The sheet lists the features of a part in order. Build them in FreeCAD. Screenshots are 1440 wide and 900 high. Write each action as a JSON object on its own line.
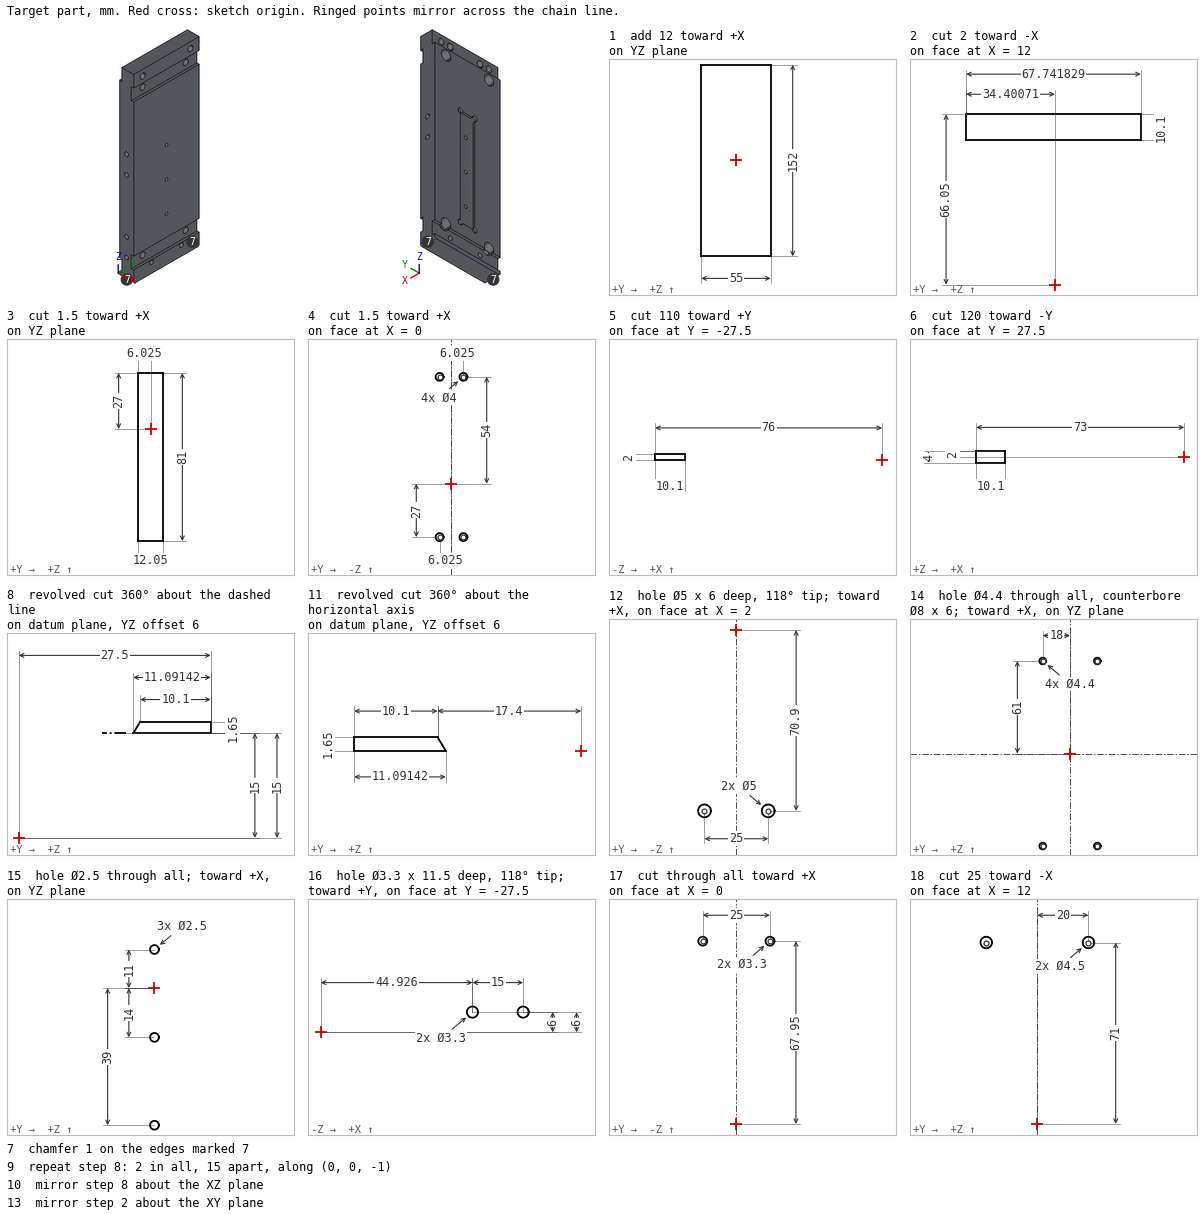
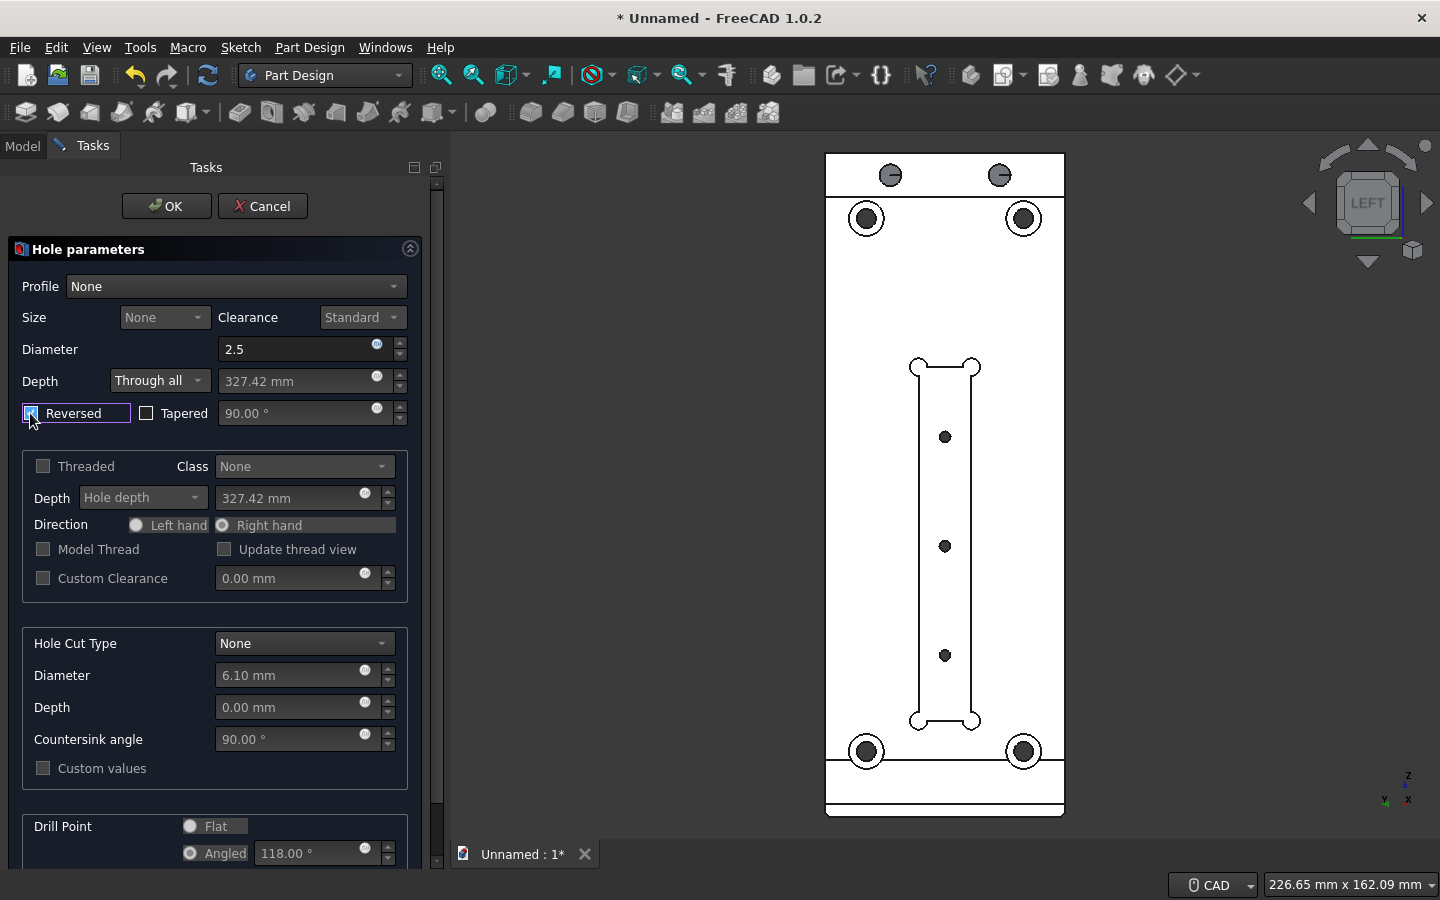
{"action": "left_click", "coordinate": [167, 206]}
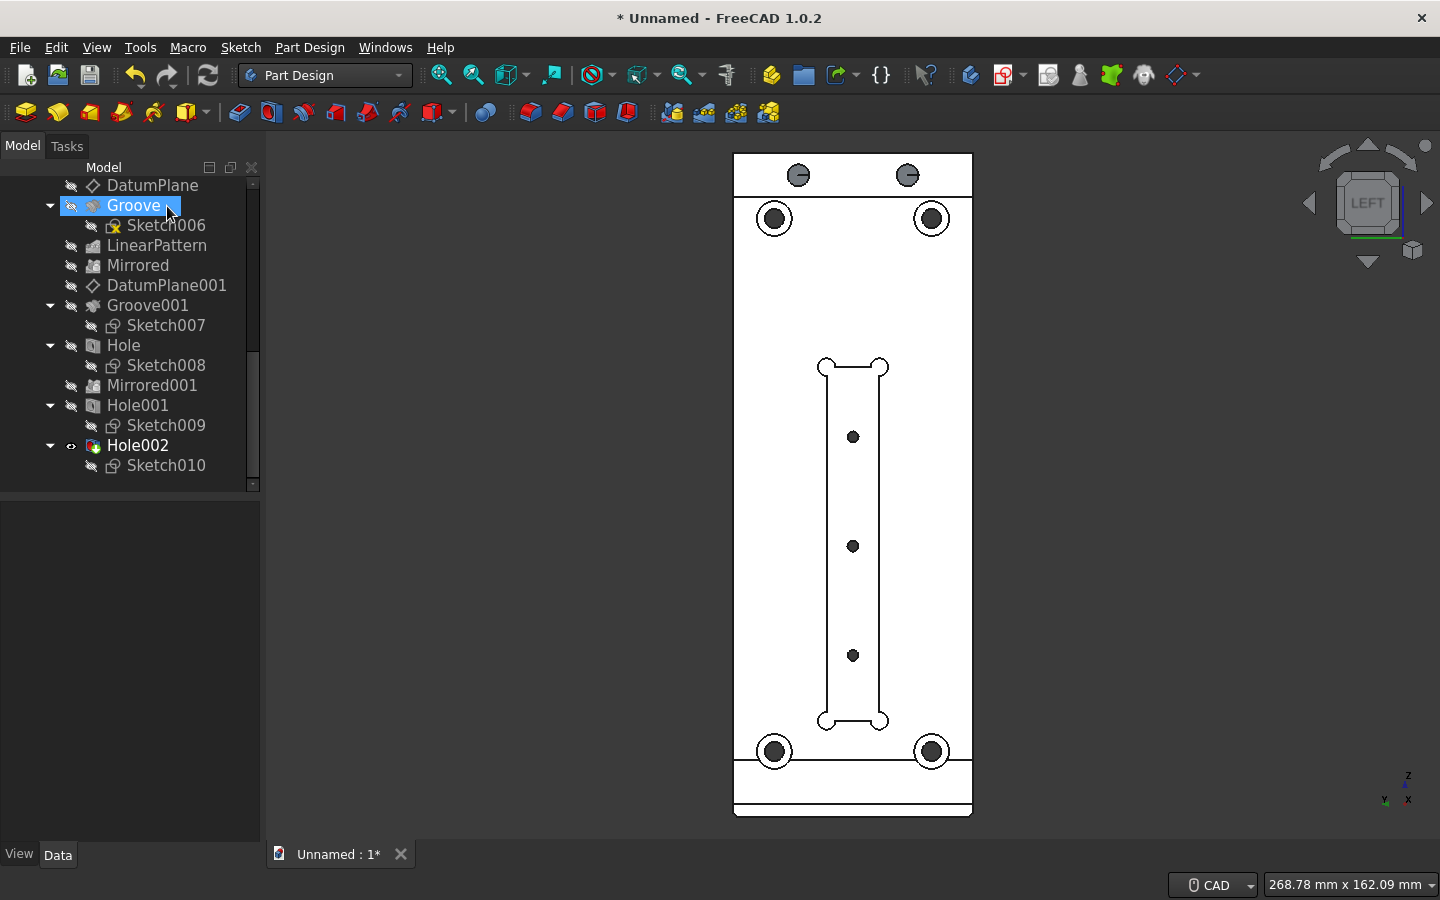
{"action": "key", "text": "0"}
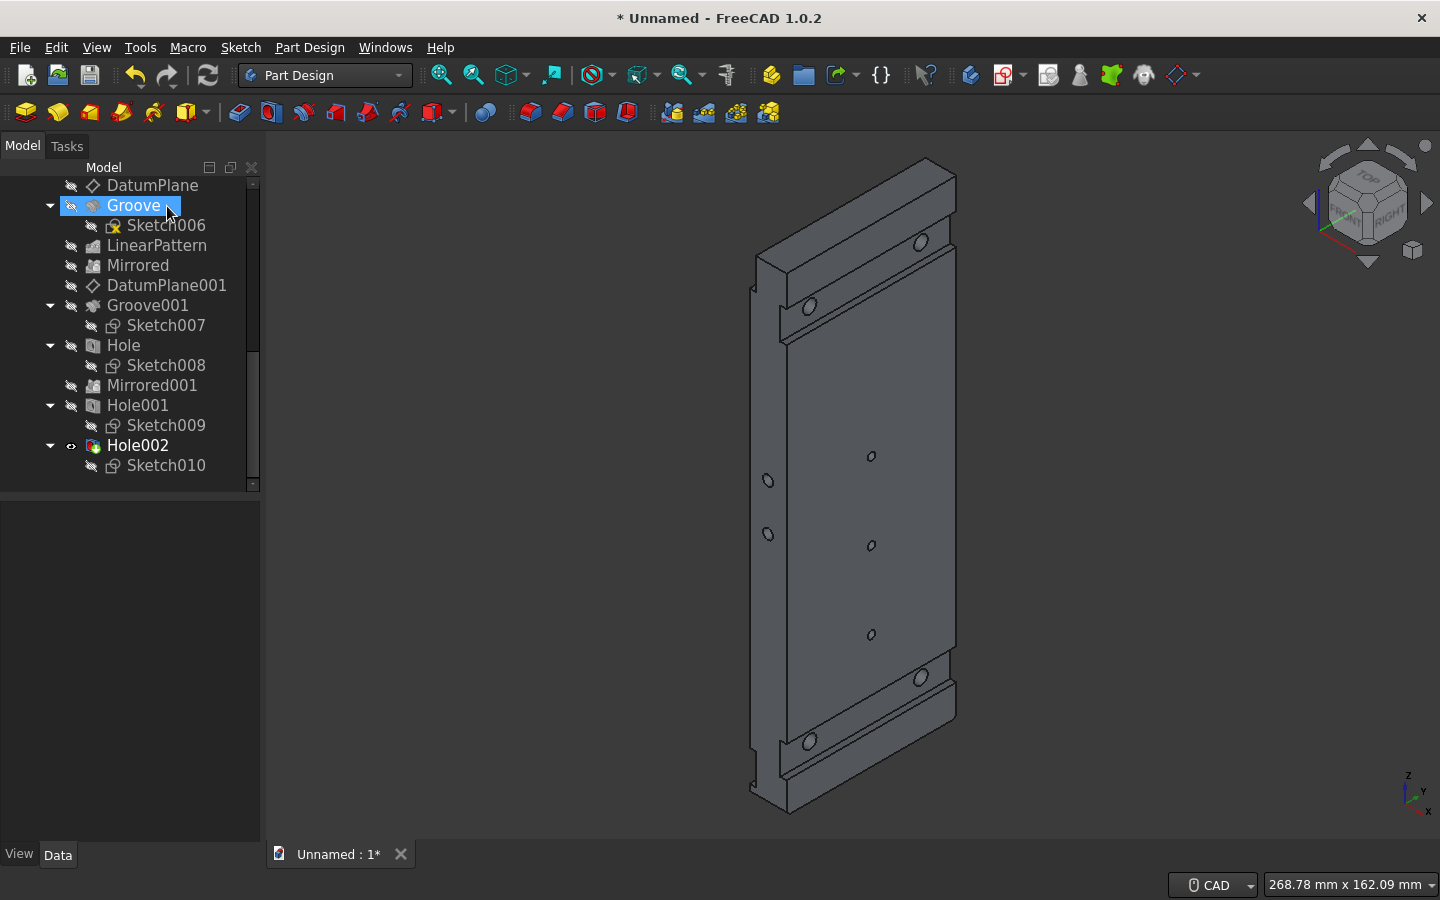
{"action": "left_click", "coordinate": [768, 685]}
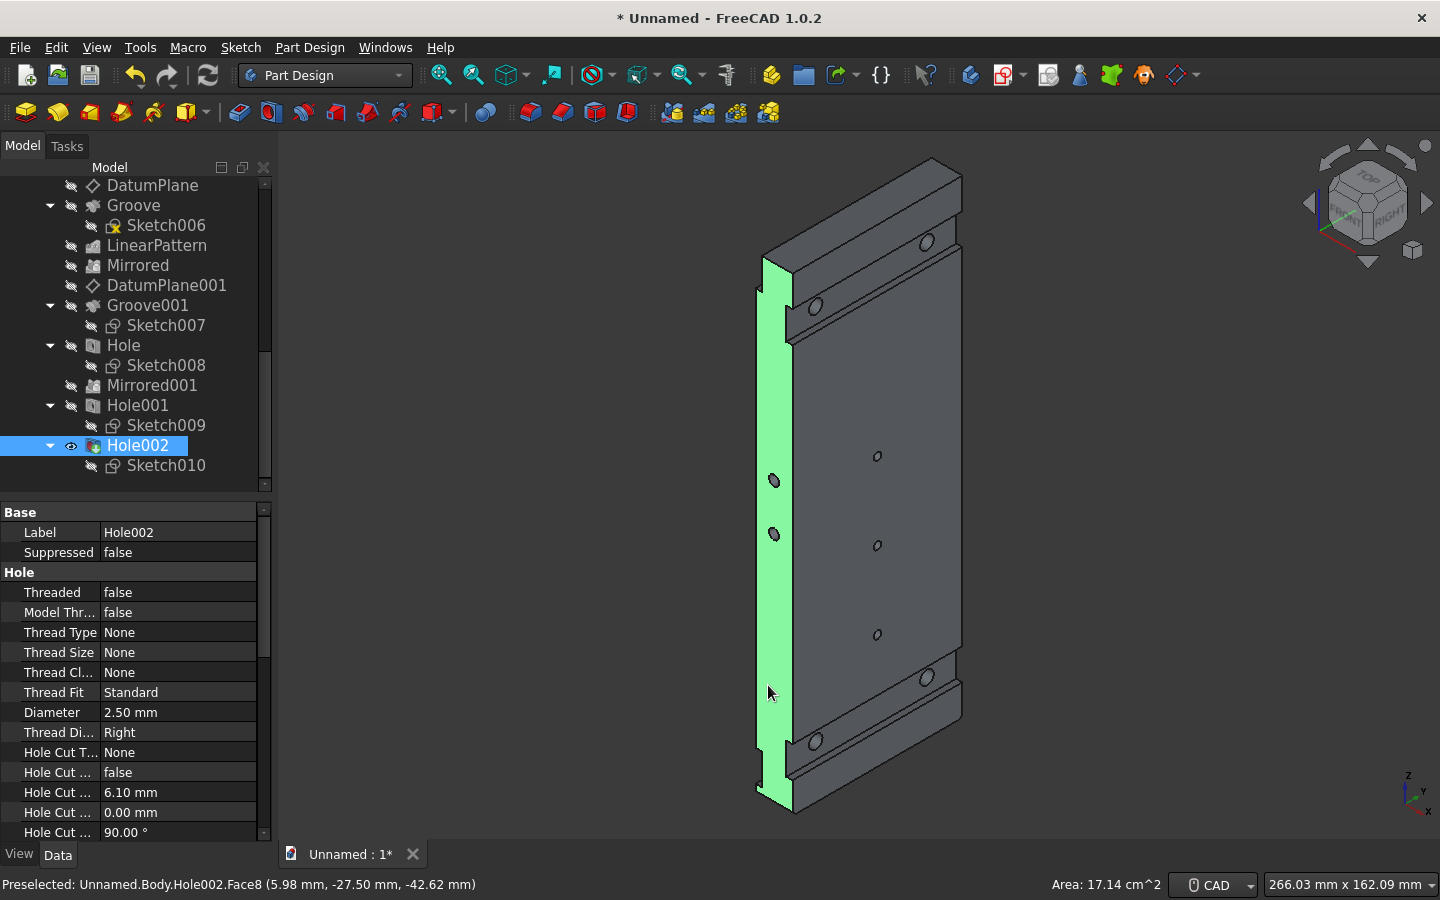
{"action": "left_click", "coordinate": [1004, 76]}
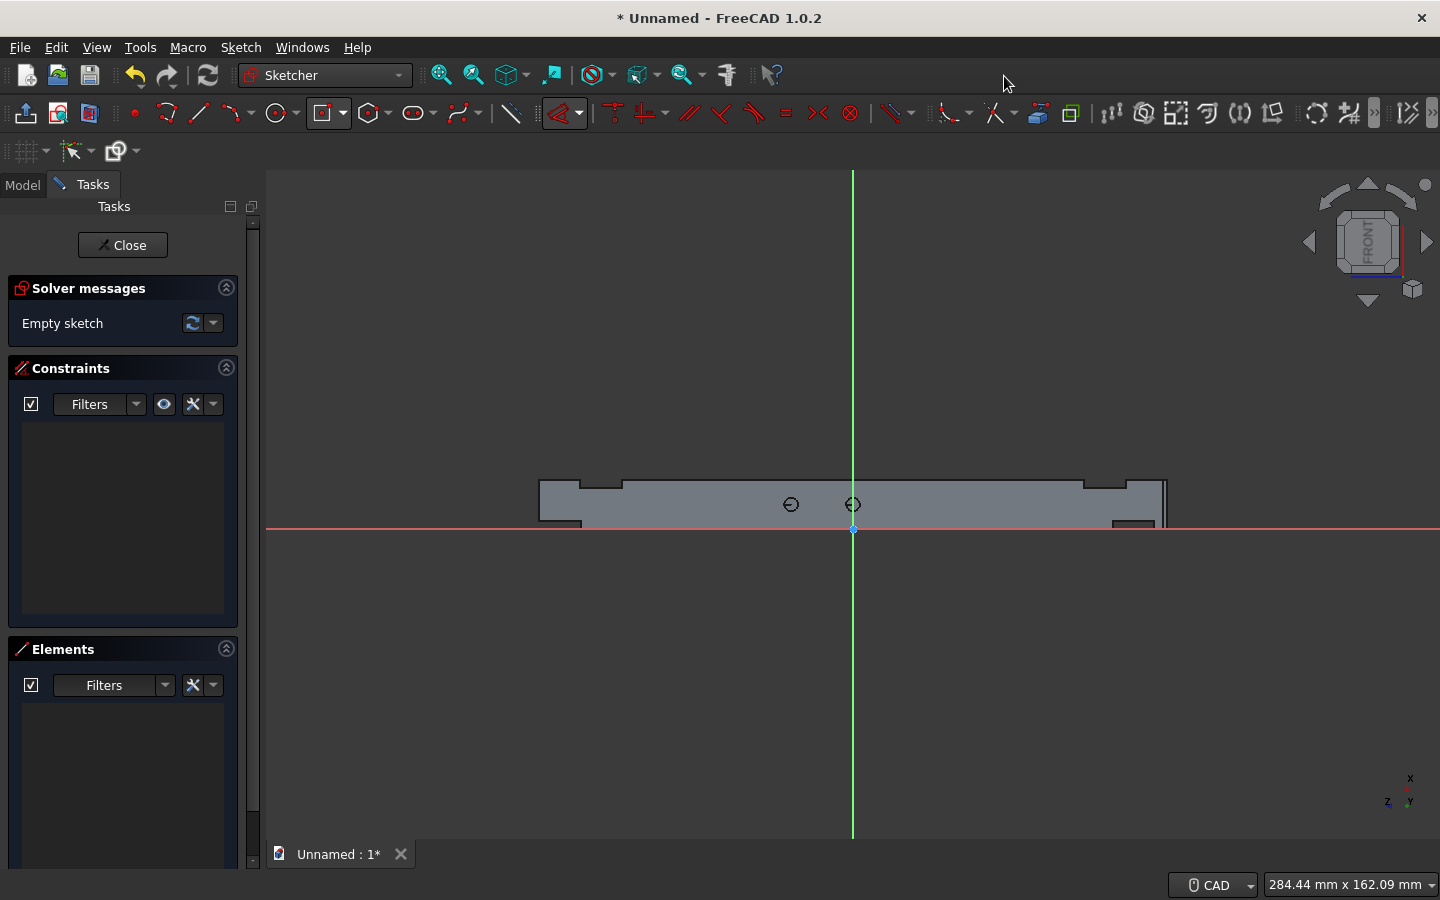
{"action": "scroll", "coordinate": [1105, 505], "scroll_direction": "up", "scroll_amount": 11}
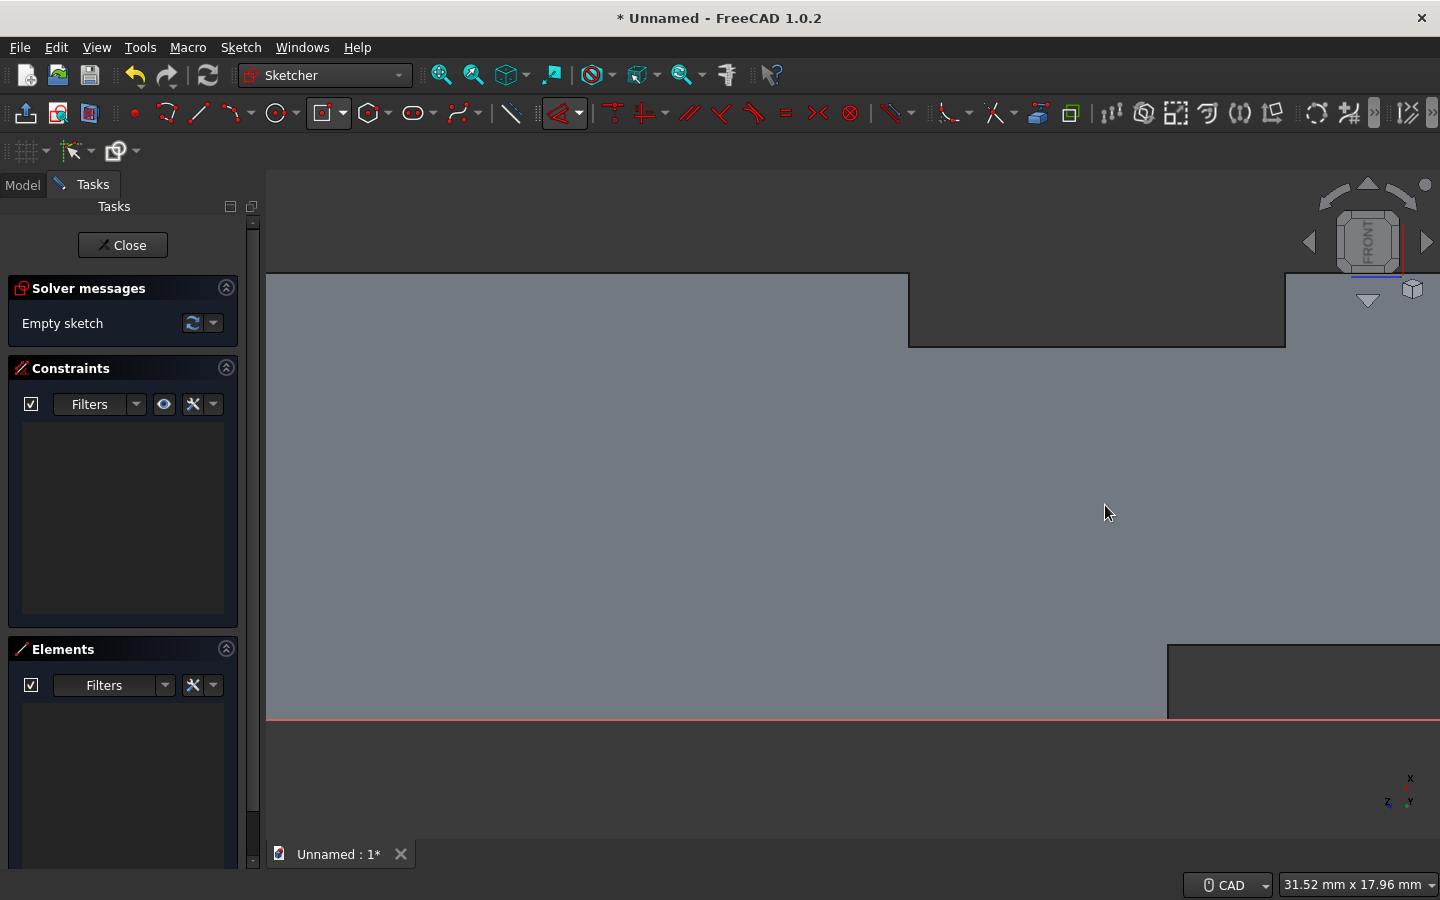
{"action": "left_click", "coordinate": [276, 114]}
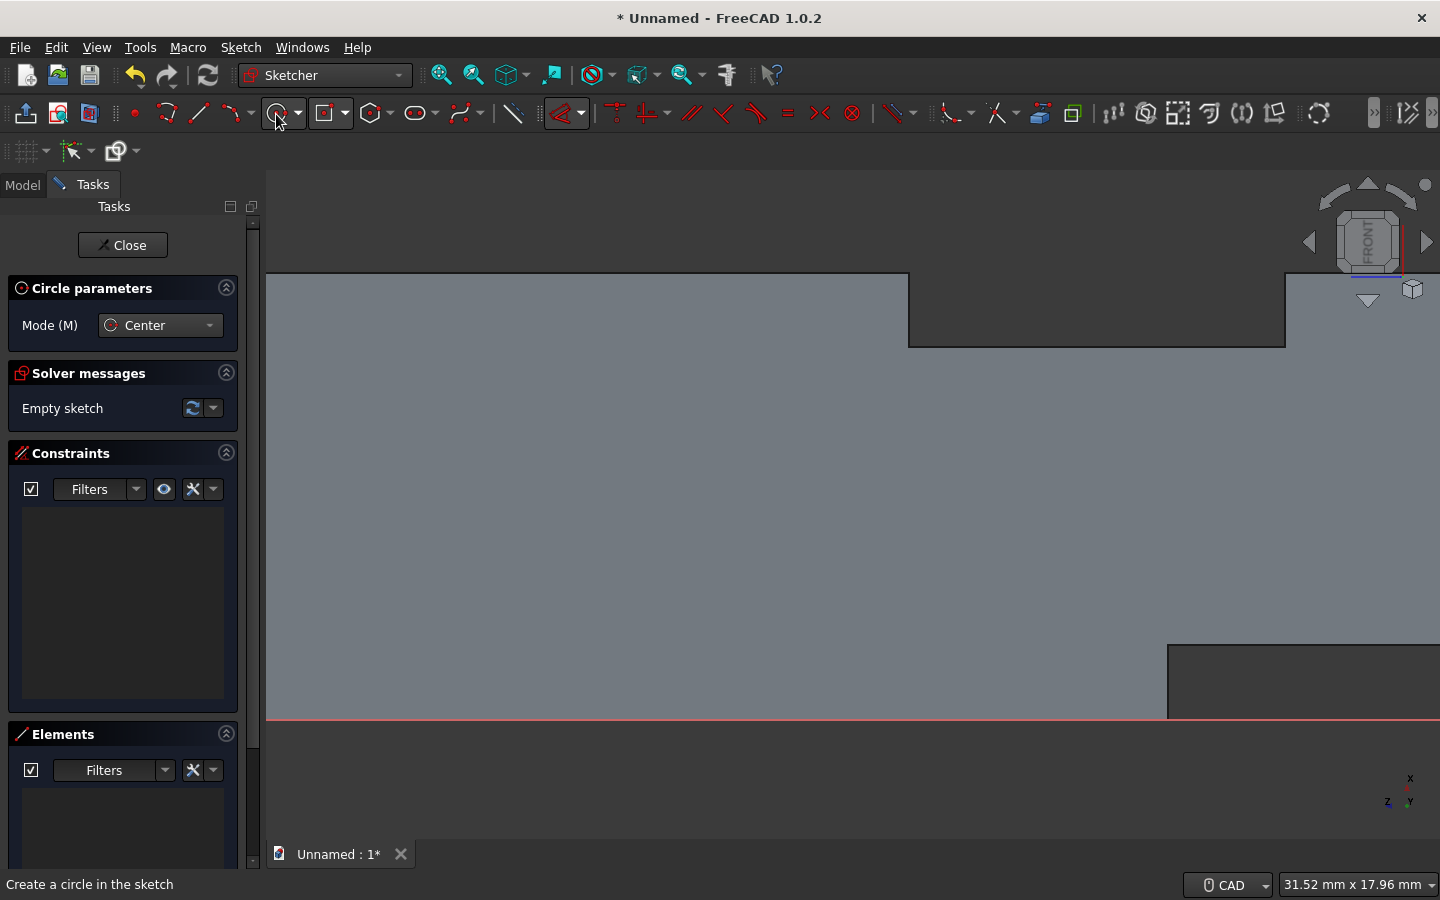
{"action": "left_click", "coordinate": [498, 496]}
{"action": "mouse_move", "coordinate": [542, 453]}